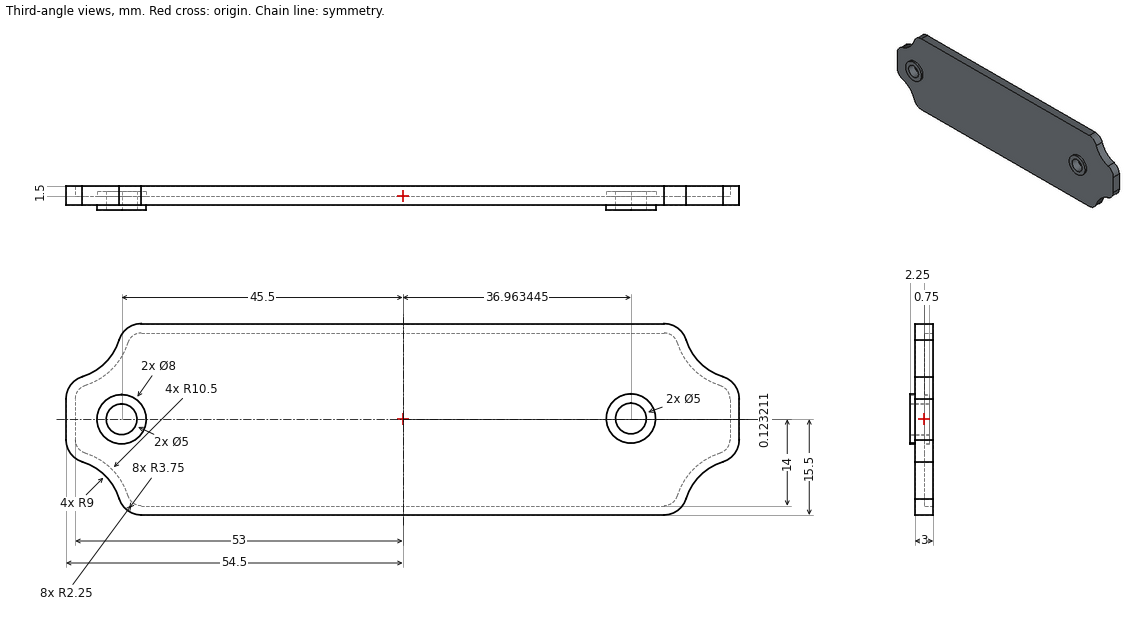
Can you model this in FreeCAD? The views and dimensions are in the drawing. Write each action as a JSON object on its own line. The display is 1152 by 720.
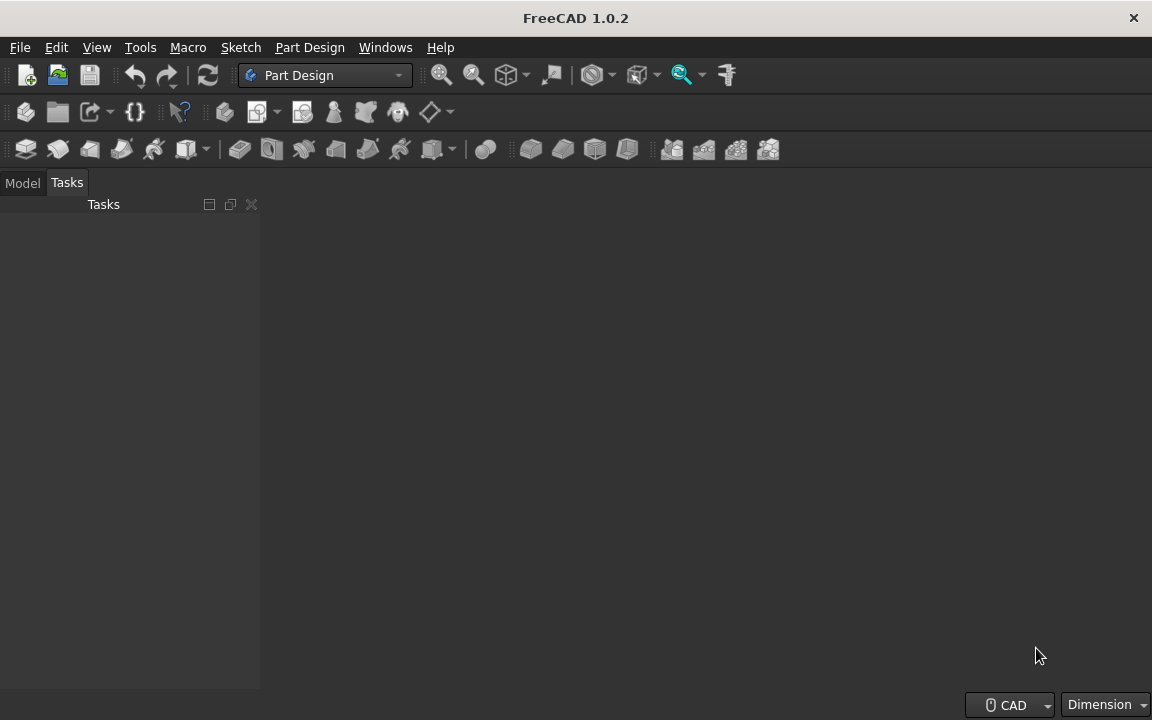
{"action": "left_click", "coordinate": [26, 76]}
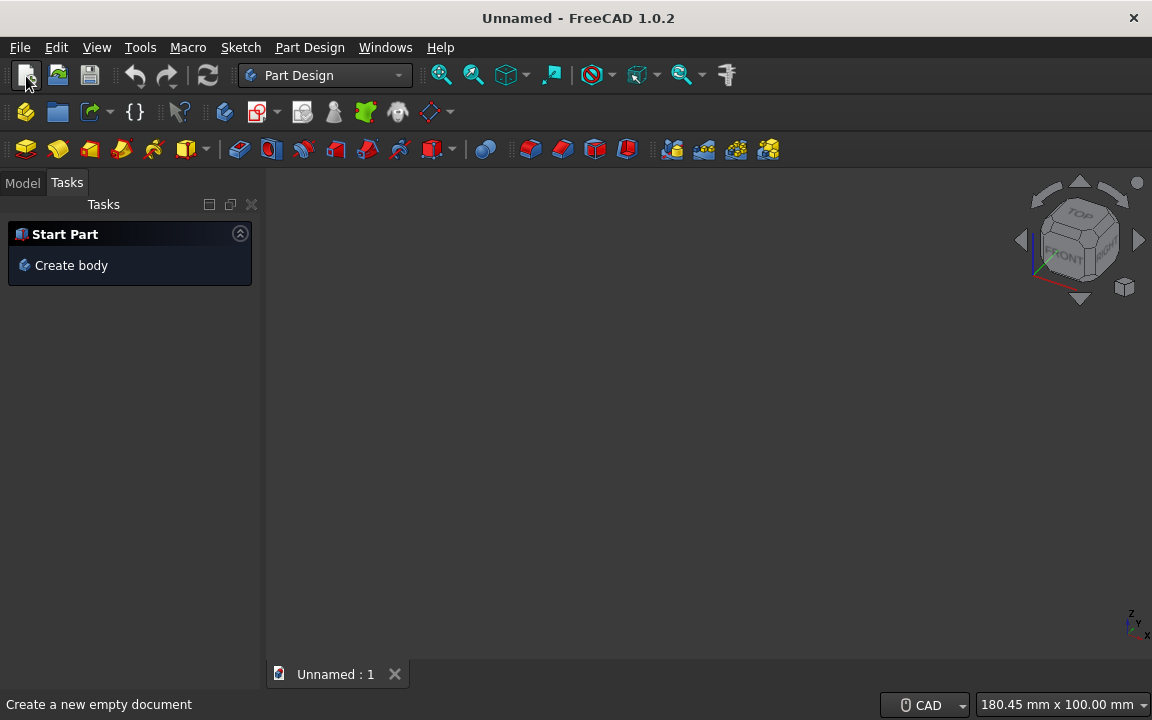
{"action": "left_click", "coordinate": [258, 112]}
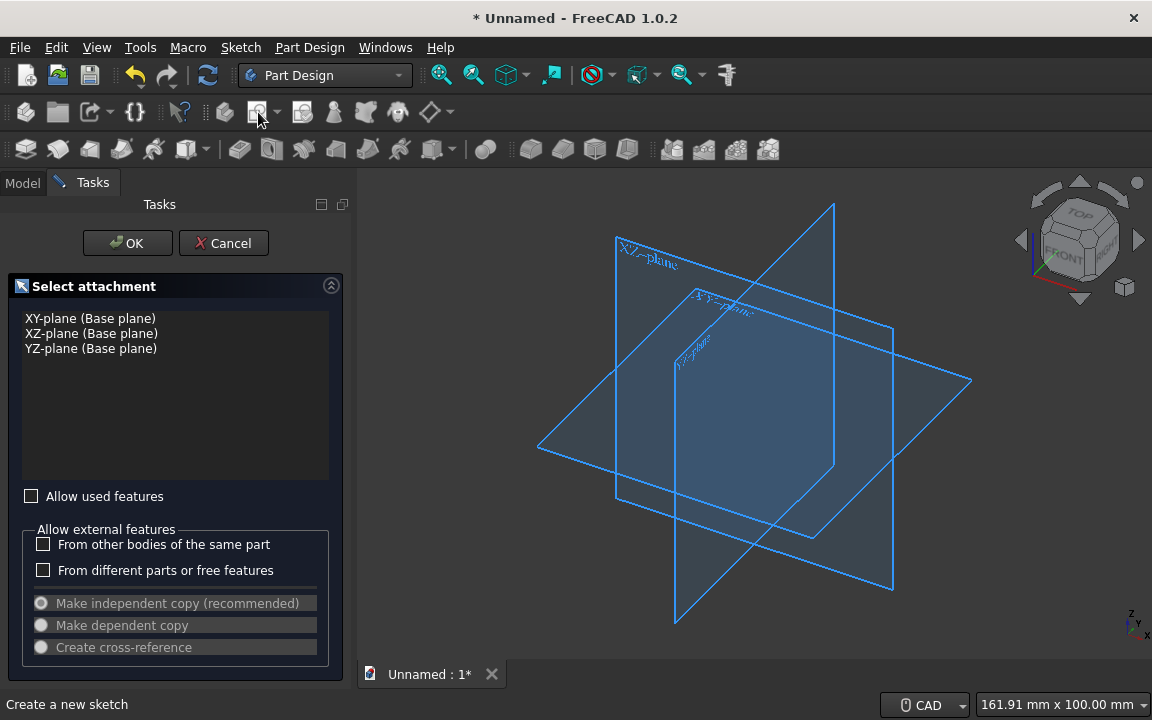
{"action": "left_click", "coordinate": [82, 334]}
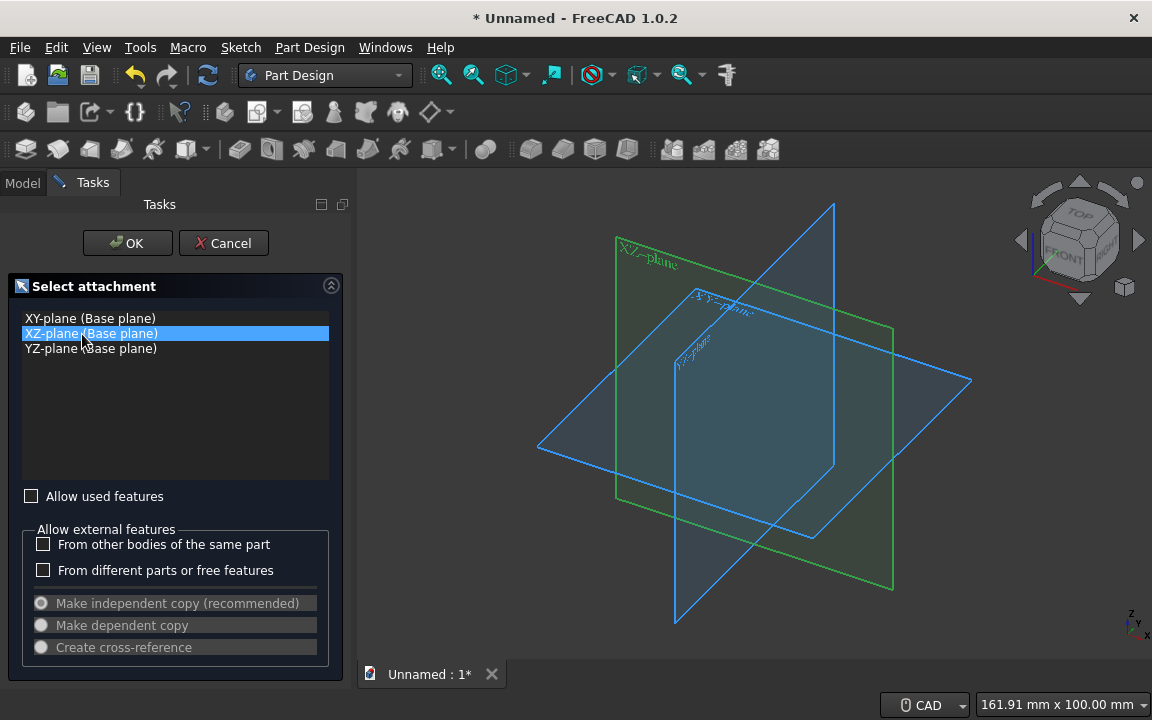
{"action": "left_click", "coordinate": [128, 243]}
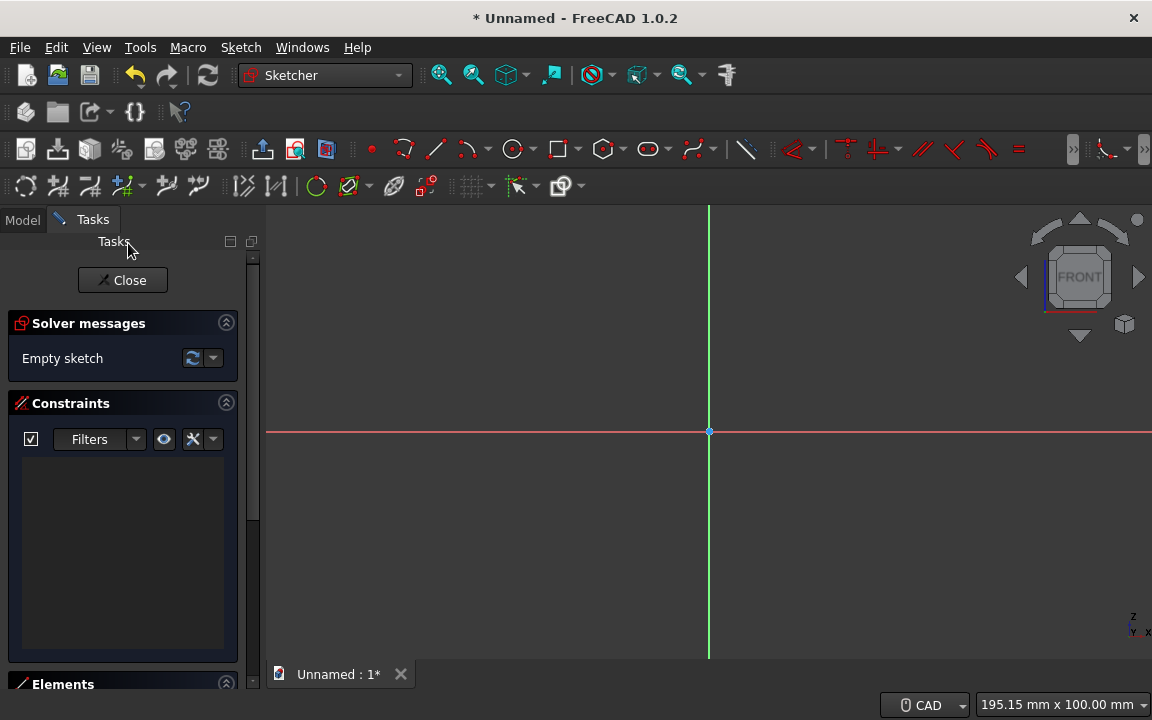
{"action": "left_click", "coordinate": [436, 150]}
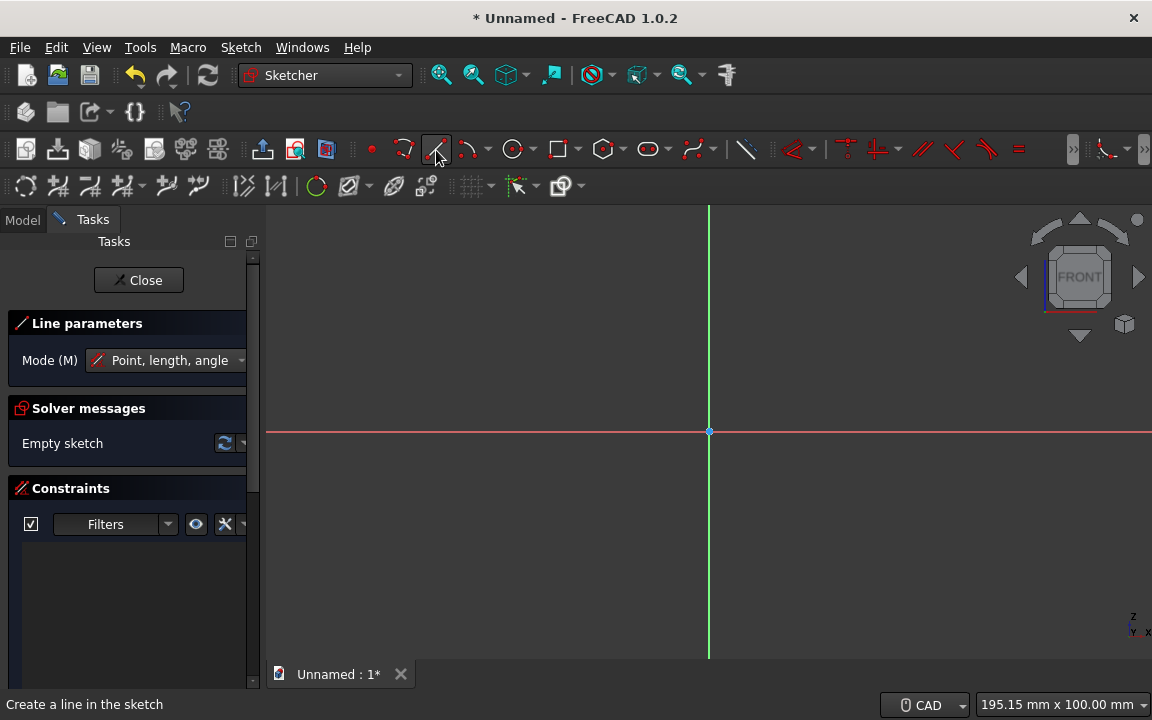
{"action": "left_click", "coordinate": [901, 502]}
{"action": "left_click", "coordinate": [517, 502]}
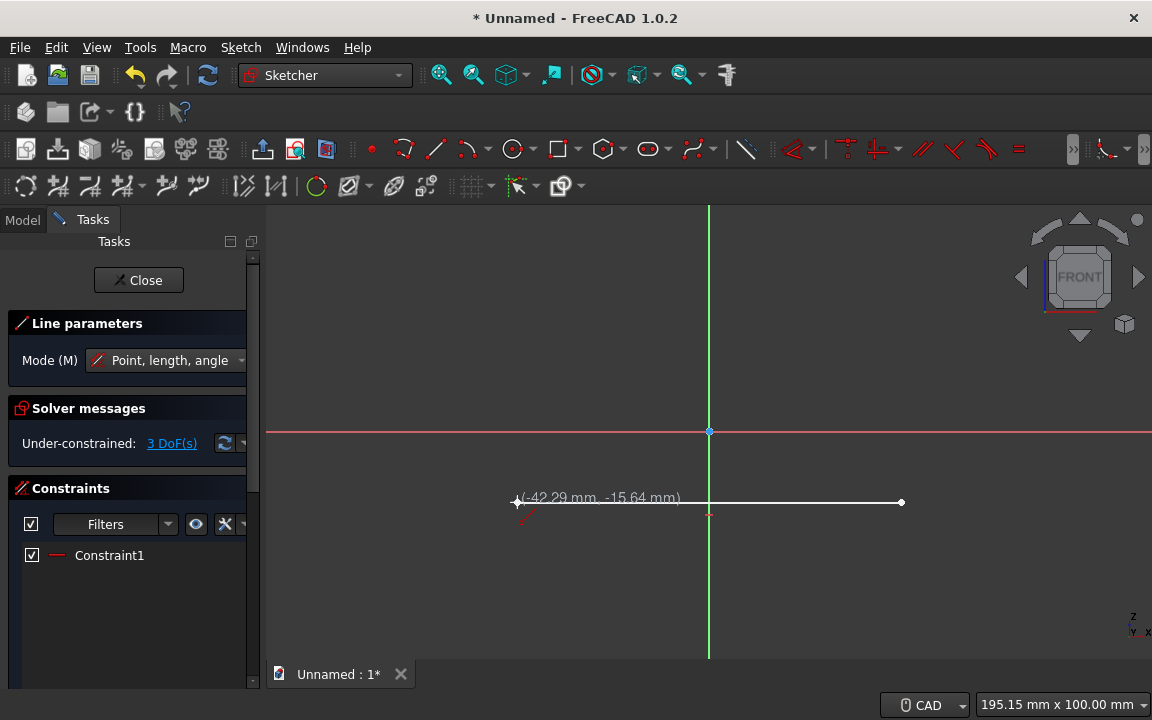
{"action": "left_click", "coordinate": [462, 447]}
{"action": "left_click", "coordinate": [462, 417]}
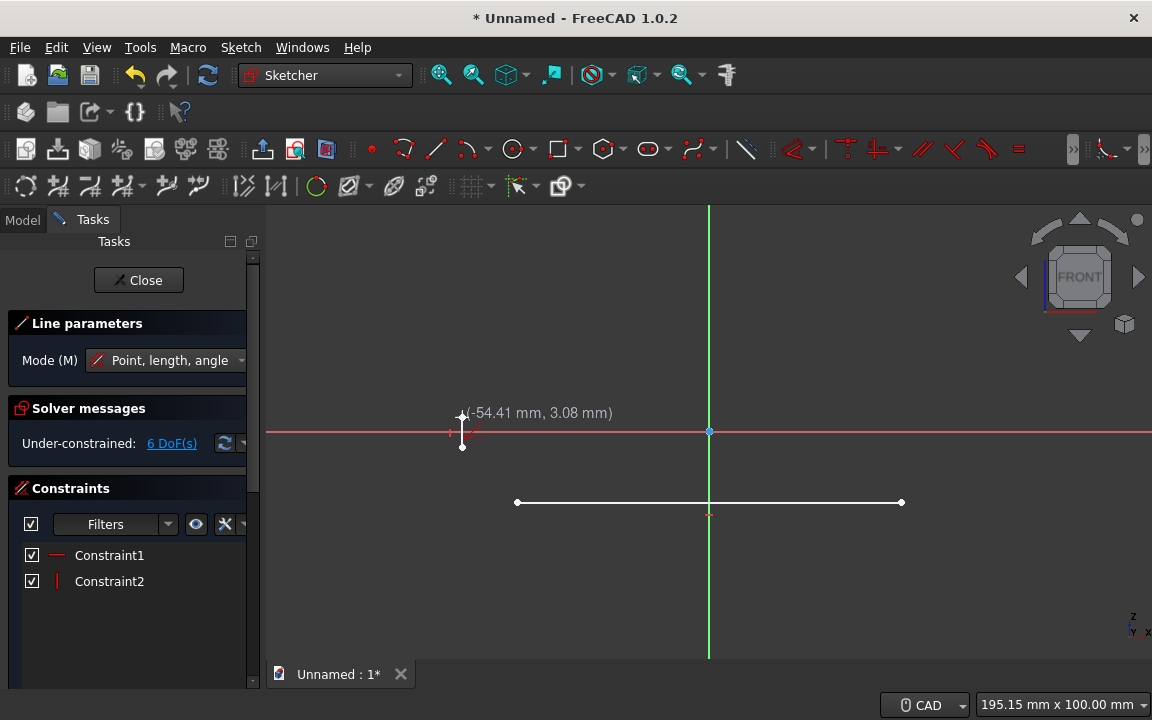
{"action": "left_click", "coordinate": [517, 362]}
{"action": "left_click", "coordinate": [901, 362]}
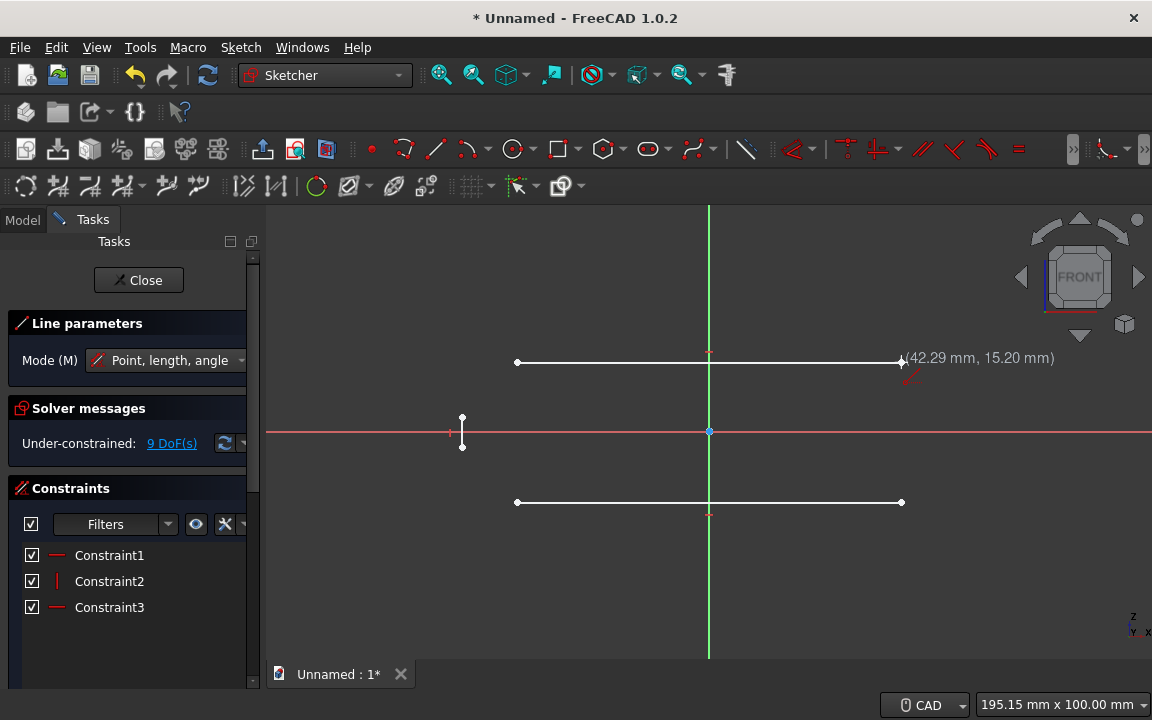
{"action": "left_click", "coordinate": [956, 417]}
{"action": "left_click", "coordinate": [956, 447]}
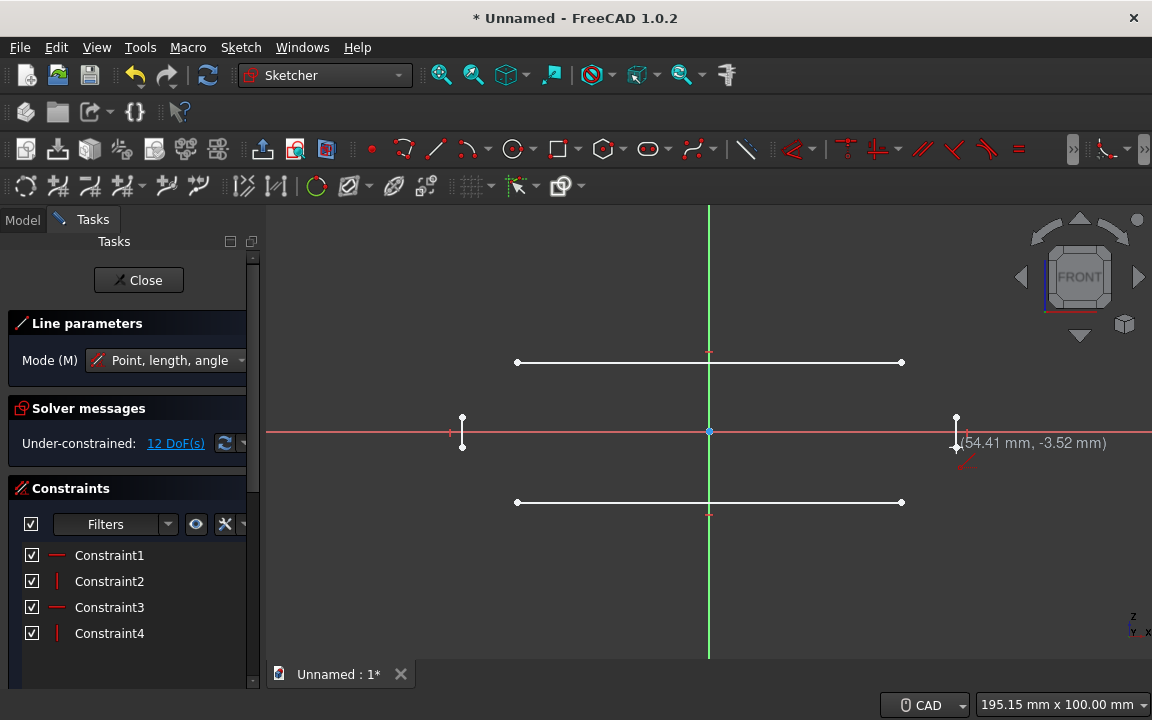
{"action": "left_click", "coordinate": [490, 150]}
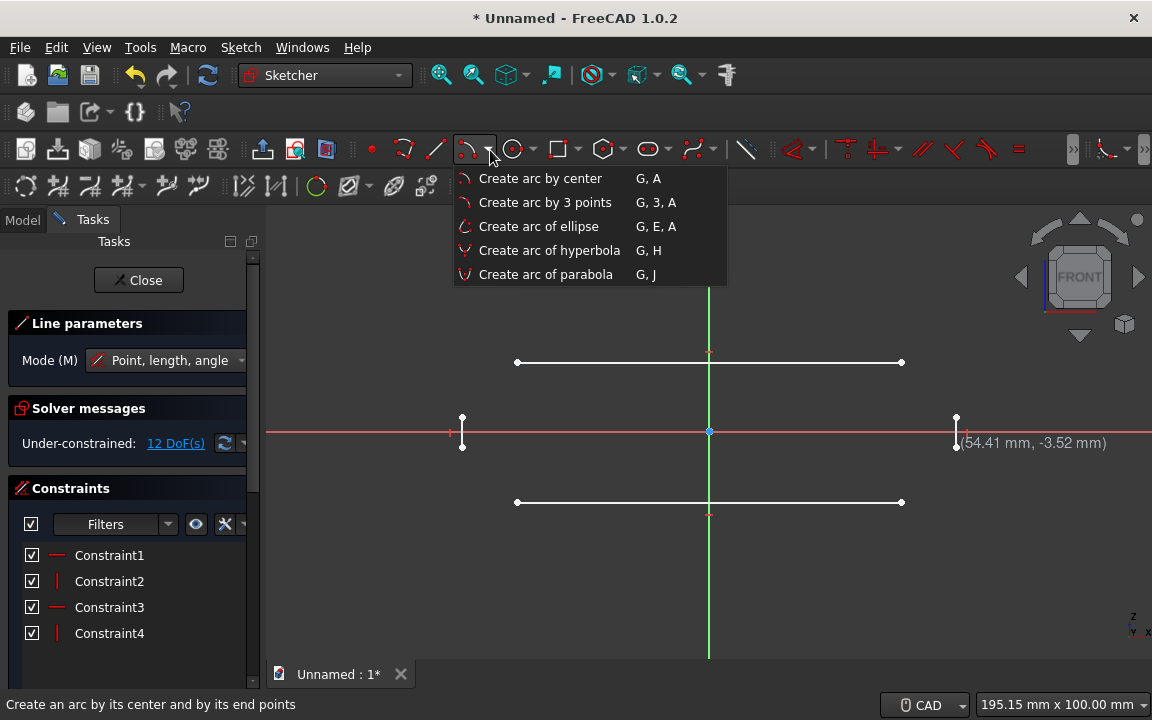
{"action": "left_click", "coordinate": [590, 202]}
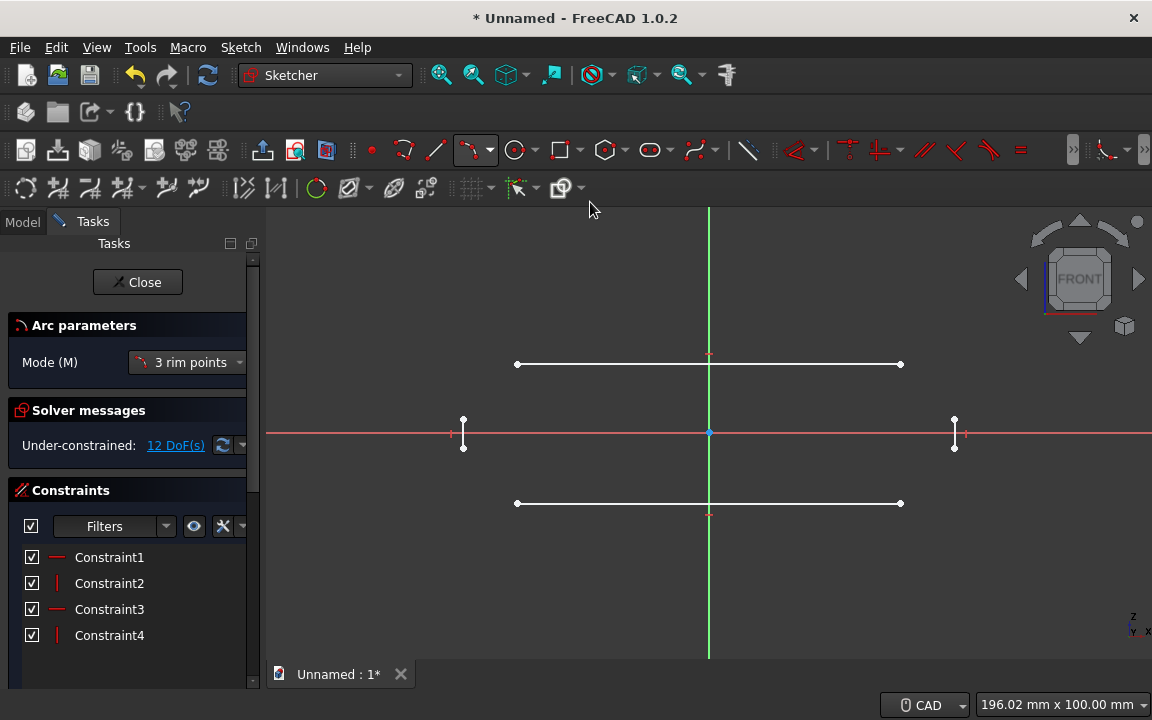
{"action": "left_click", "coordinate": [518, 504]}
{"action": "left_click", "coordinate": [502, 491]}